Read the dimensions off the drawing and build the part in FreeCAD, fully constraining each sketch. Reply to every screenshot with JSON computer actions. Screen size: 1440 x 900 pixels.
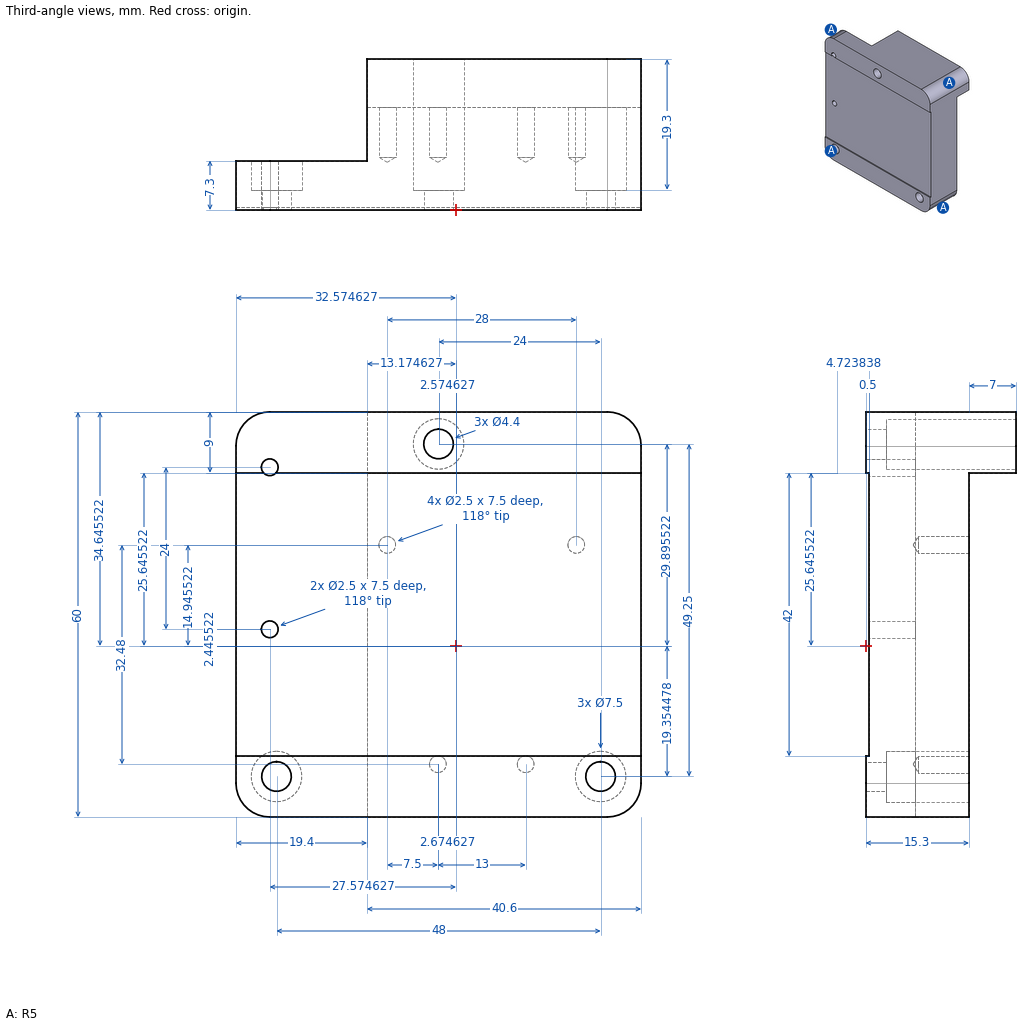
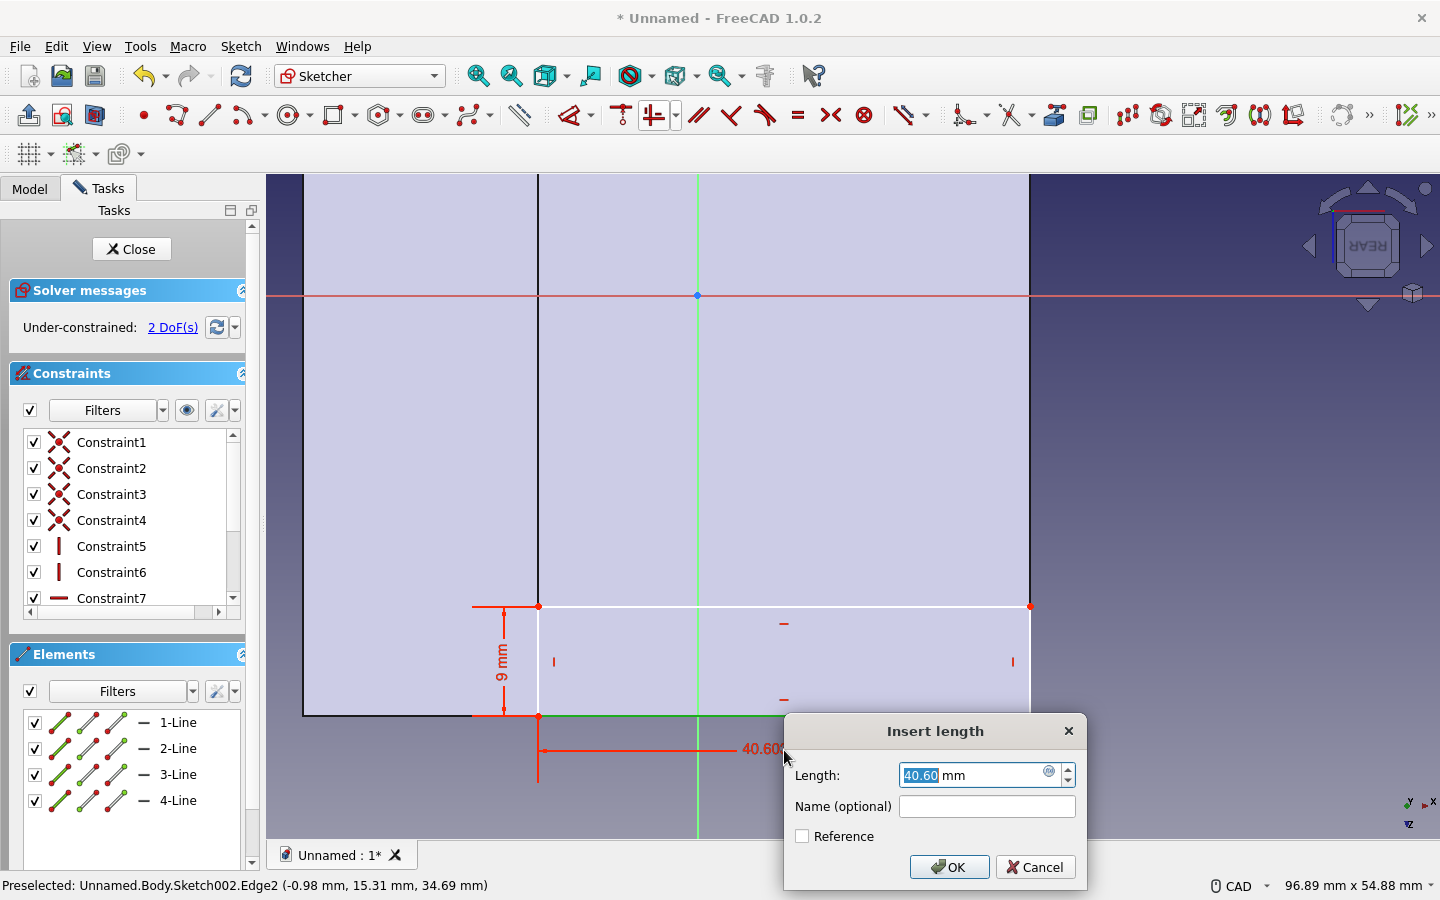
{"action": "type", "text": "40.6"}
{"action": "key", "text": "Return"}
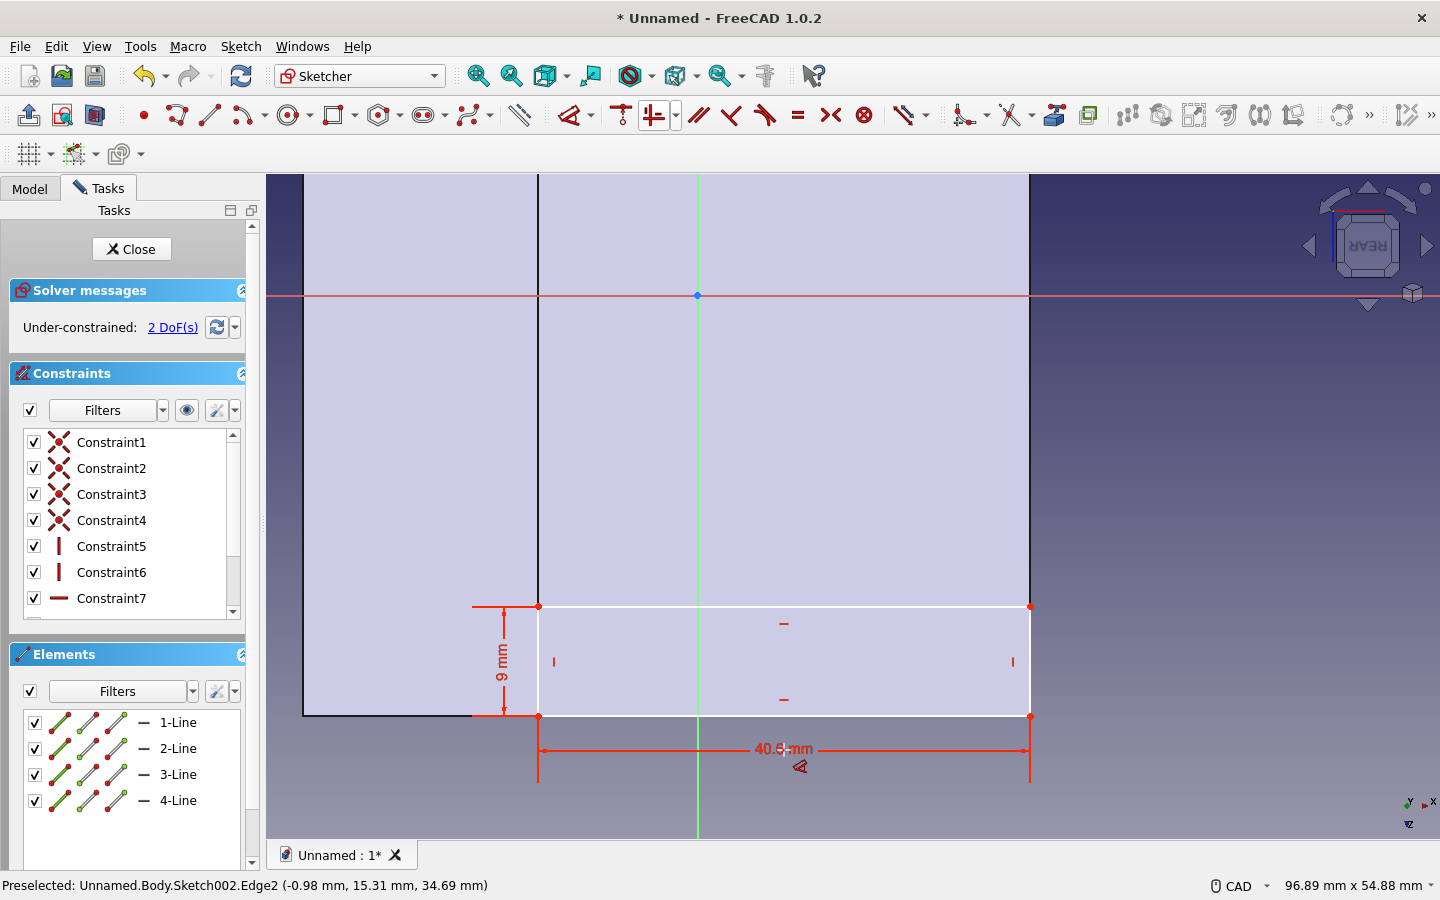
{"action": "left_click", "coordinate": [538, 607]}
{"action": "left_click", "coordinate": [618, 262]}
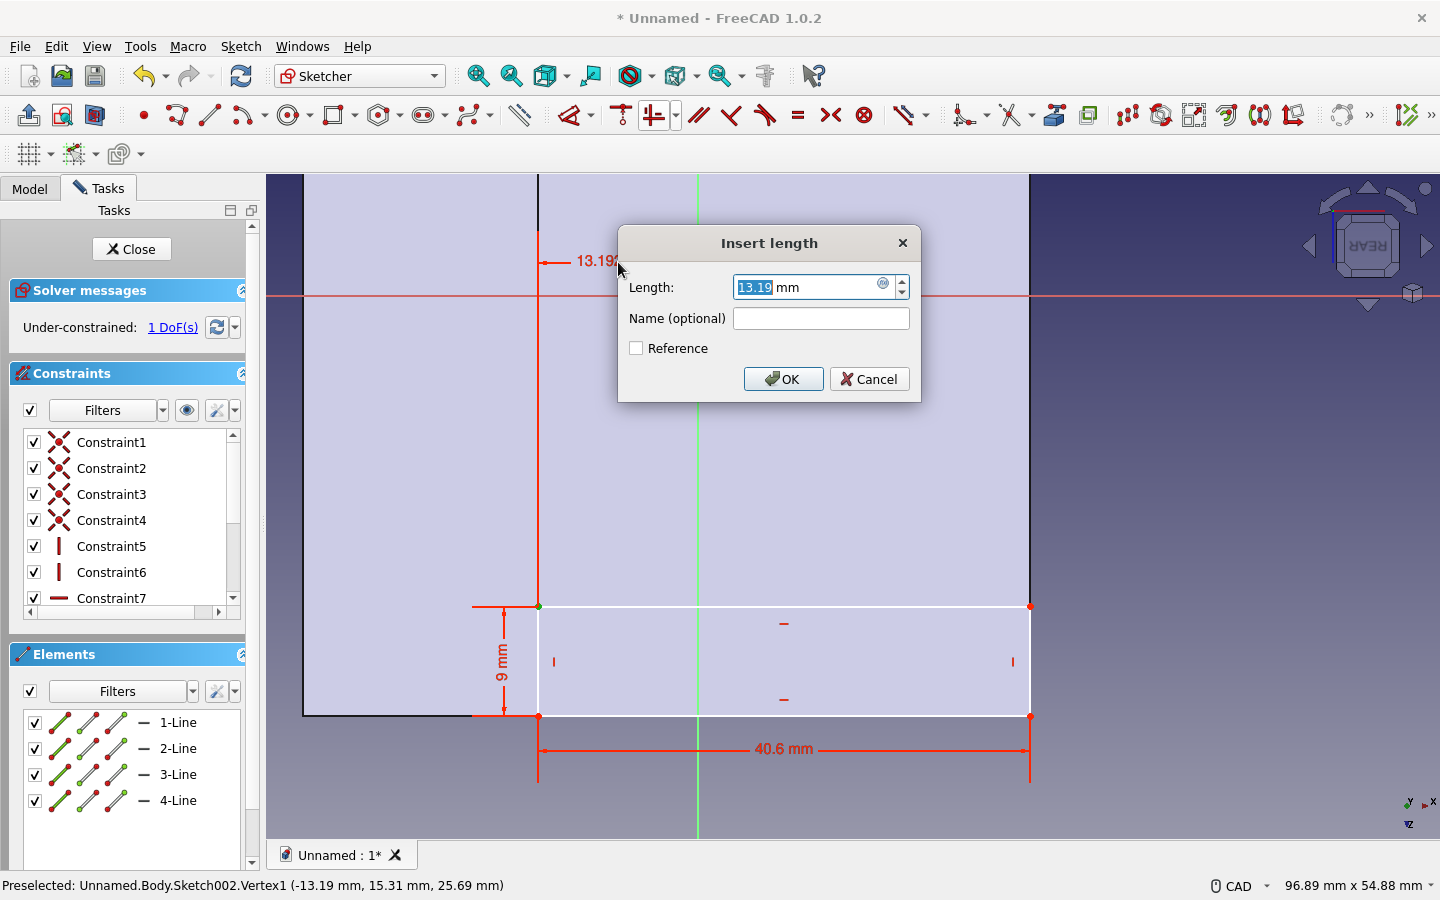
{"action": "type", "text": "13.174627"}
{"action": "key", "text": "Return"}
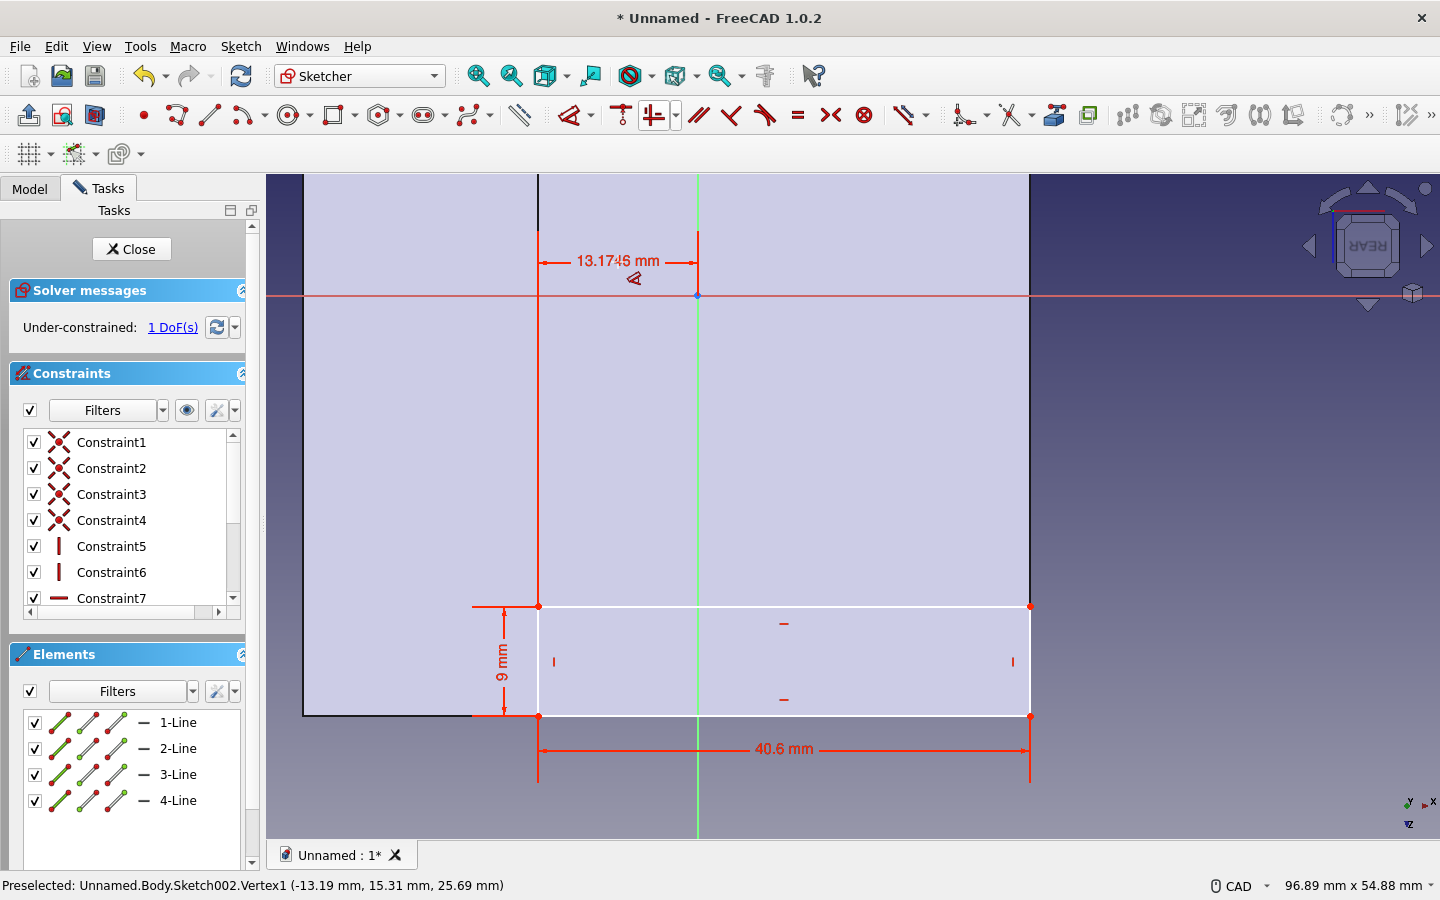
{"action": "left_click", "coordinate": [538, 607]}
{"action": "left_click", "coordinate": [504, 451]}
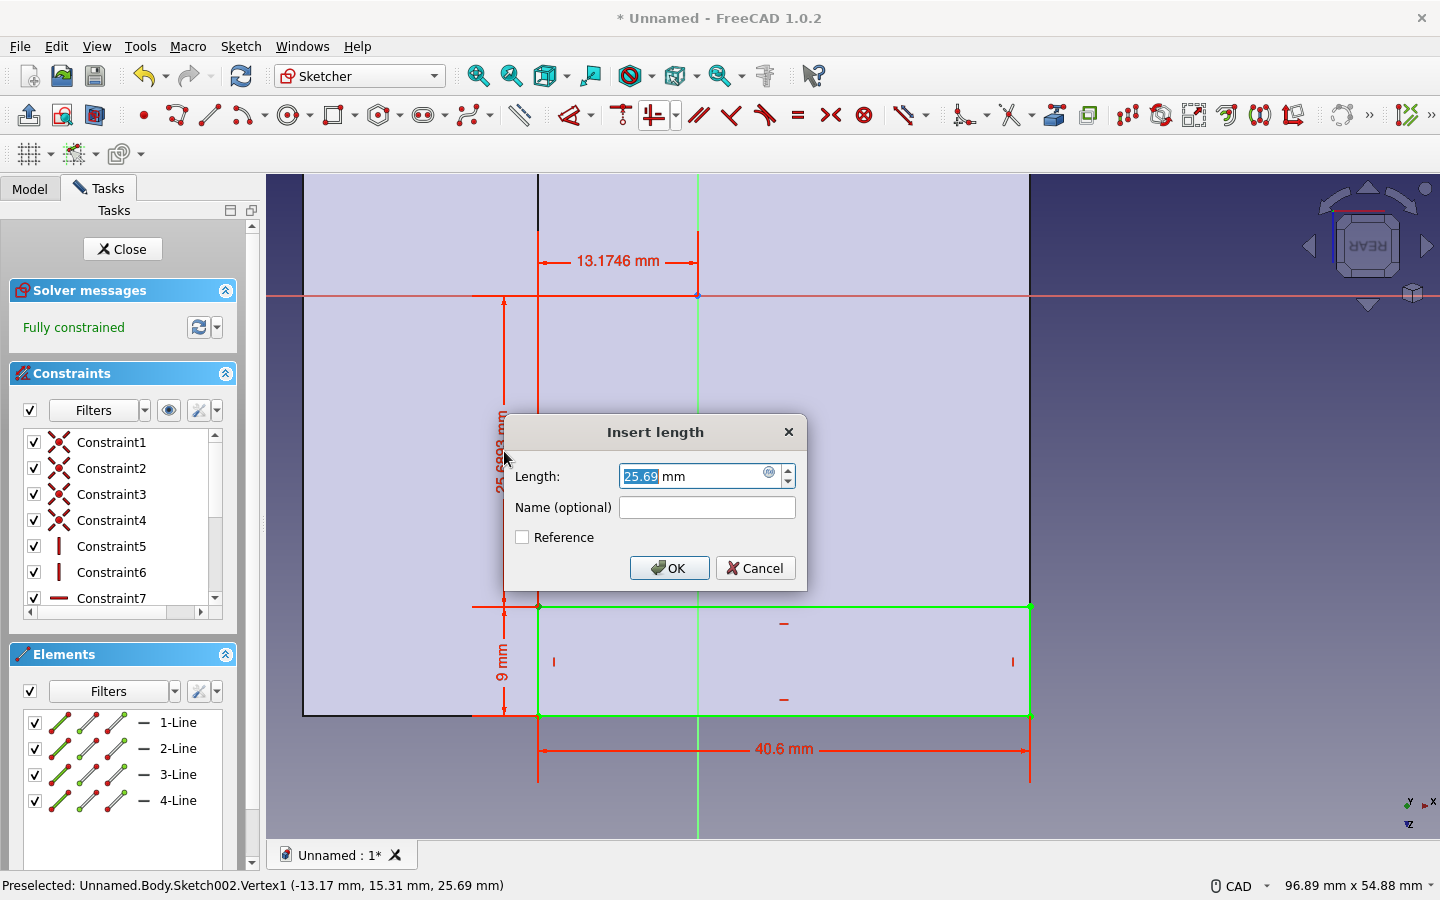
{"action": "type", "text": "25.645522"}
{"action": "key", "text": "Return"}
{"action": "key", "text": "Escape"}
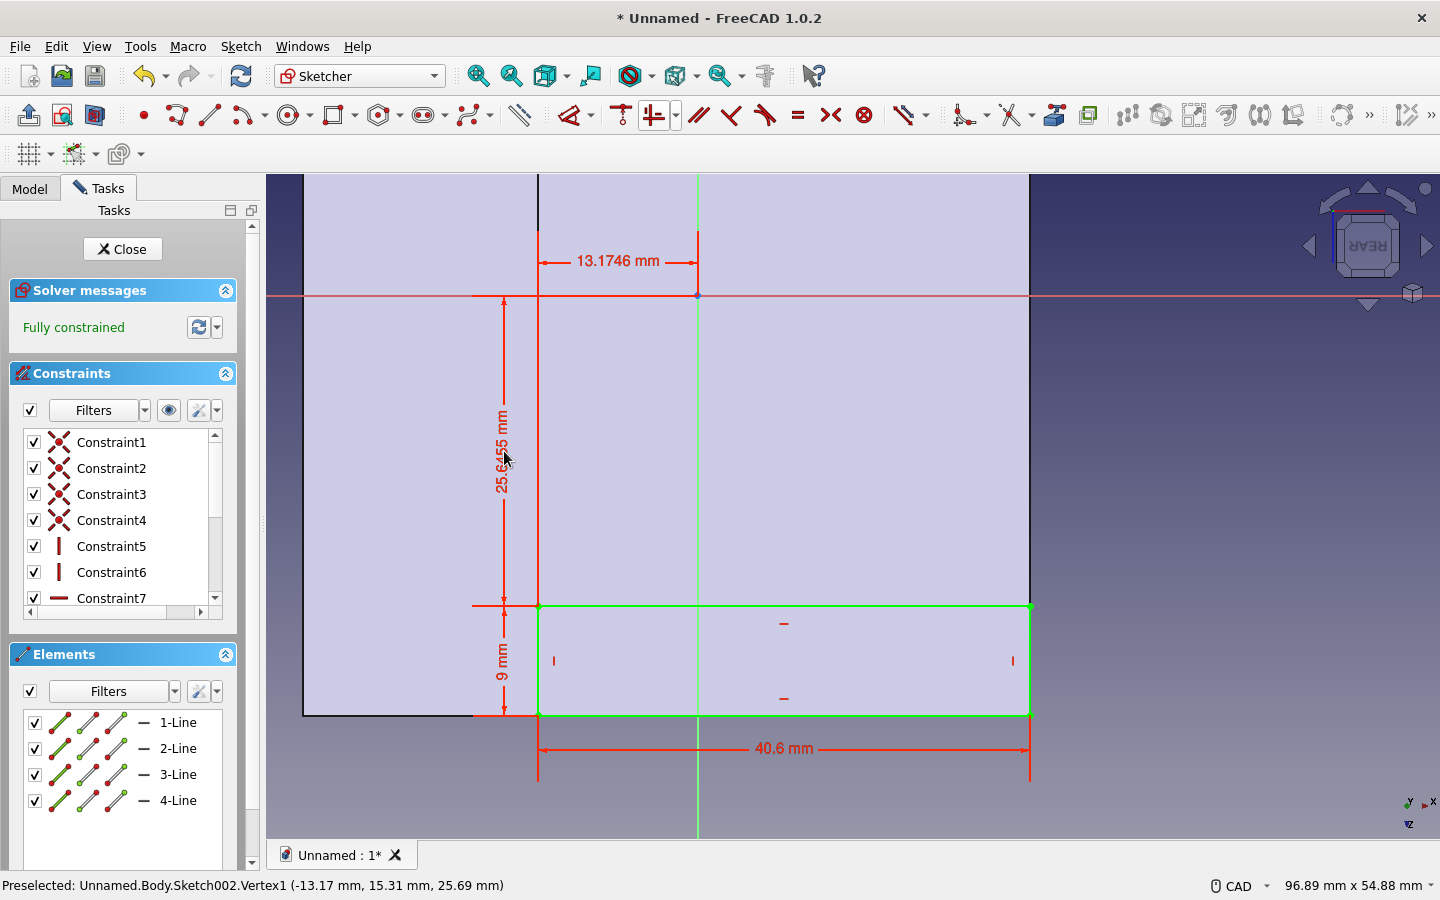
{"action": "left_click", "coordinate": [123, 249]}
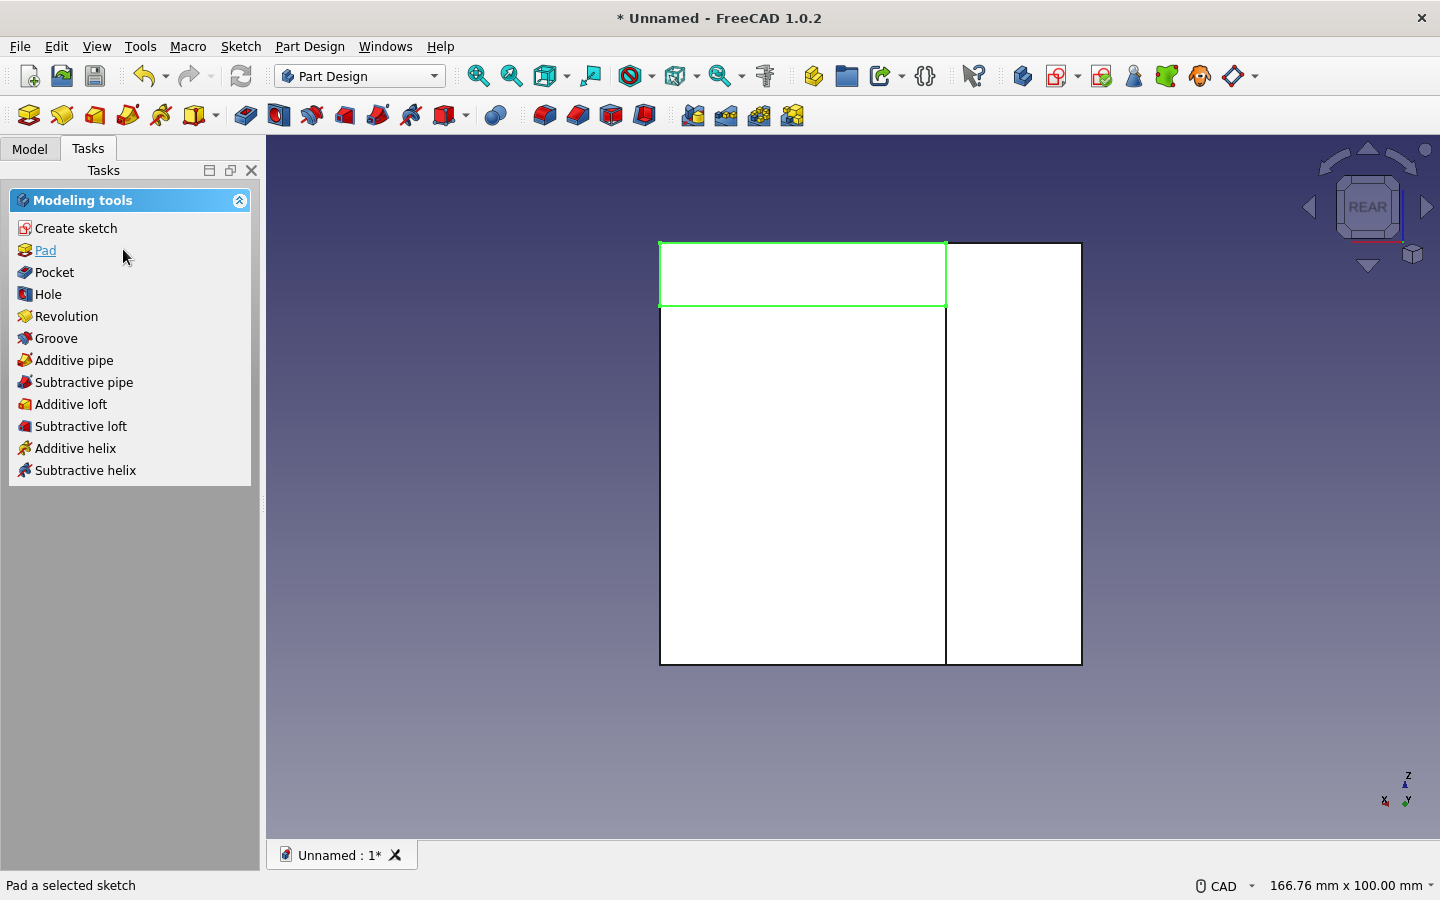
{"action": "left_click", "coordinate": [29, 116]}